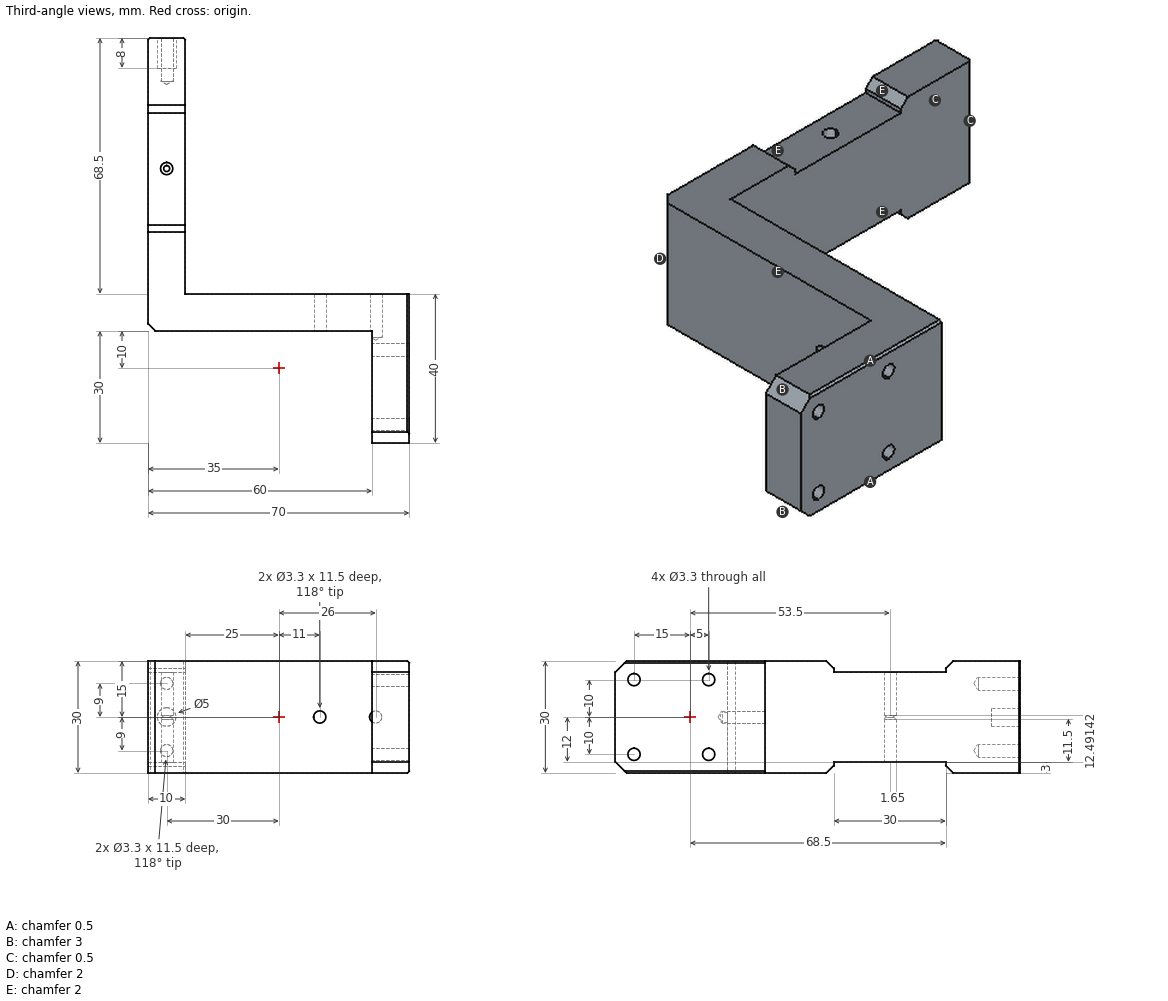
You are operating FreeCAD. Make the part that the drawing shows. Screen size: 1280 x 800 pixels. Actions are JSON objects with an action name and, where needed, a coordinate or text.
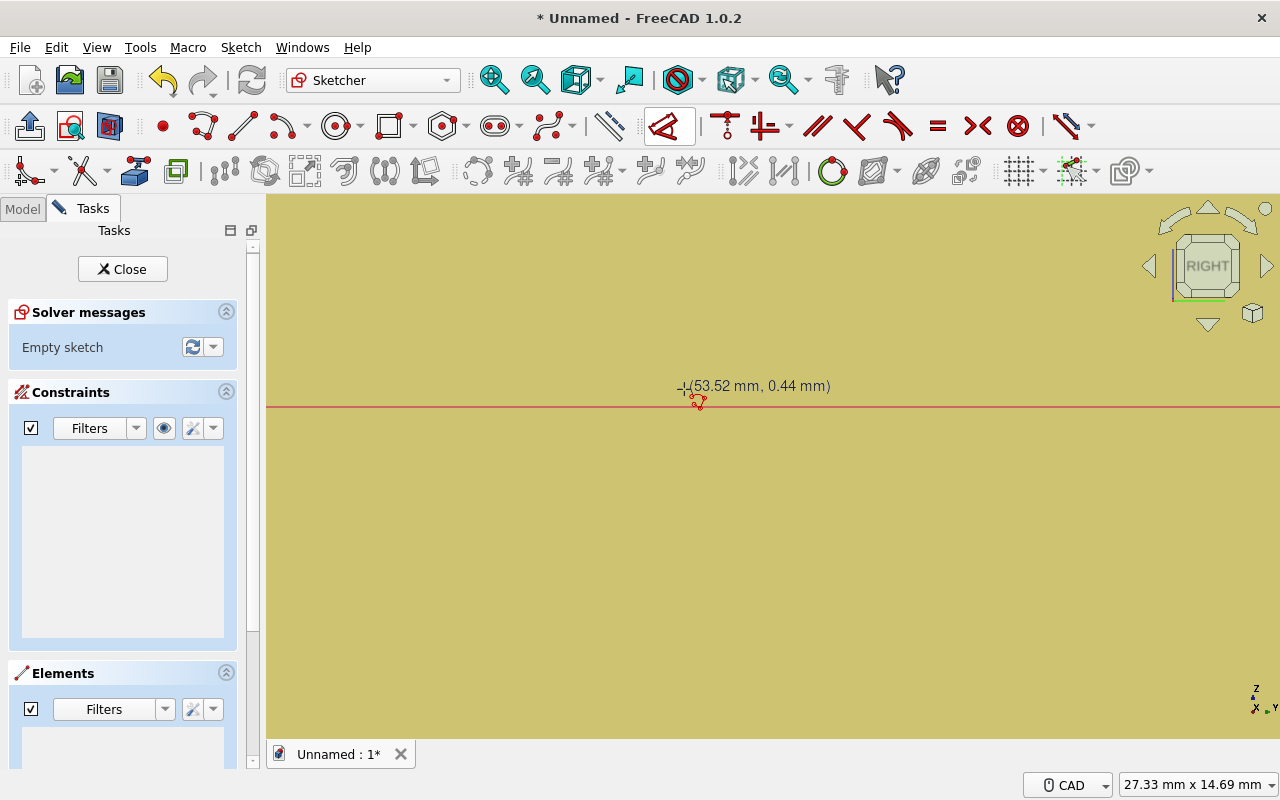
{"action": "scroll", "coordinate": [692, 392], "scroll_direction": "down", "scroll_amount": 3}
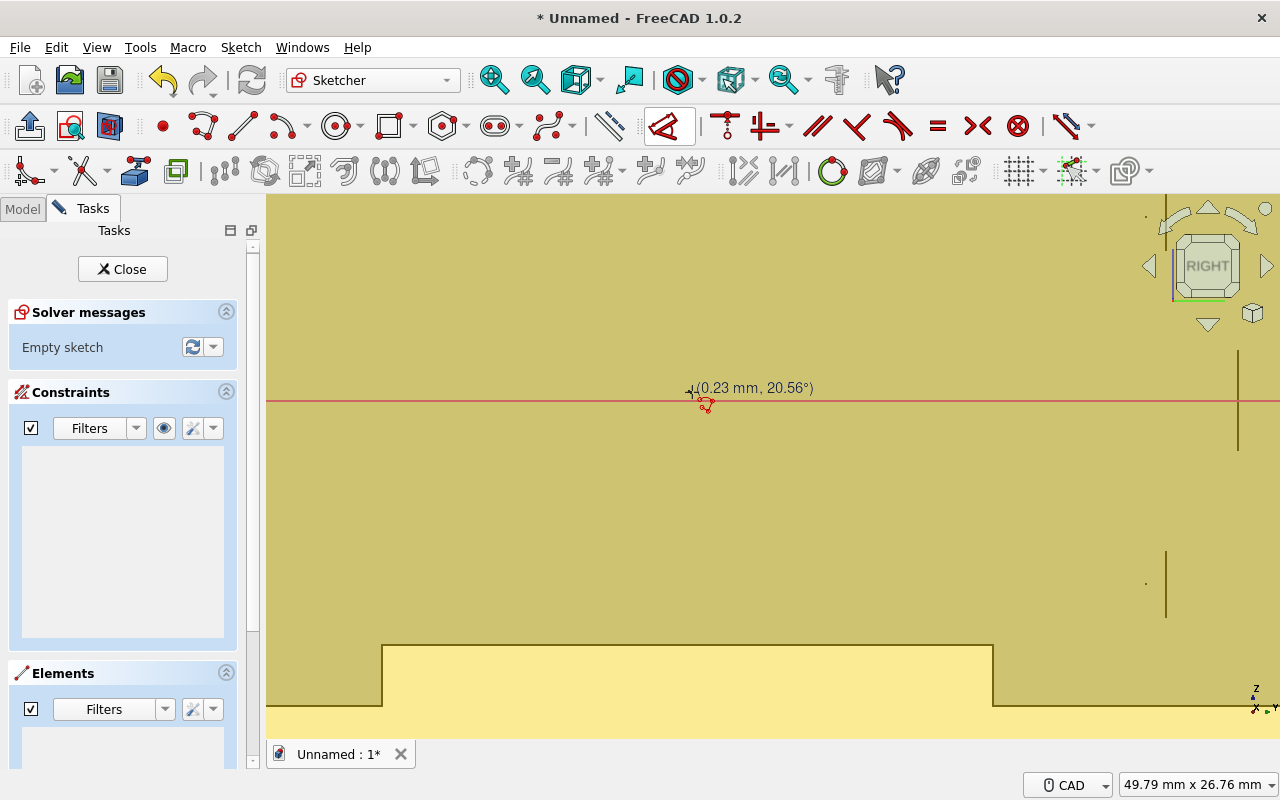
{"action": "left_click", "coordinate": [688, 645]}
{"action": "left_click", "coordinate": [721, 645]}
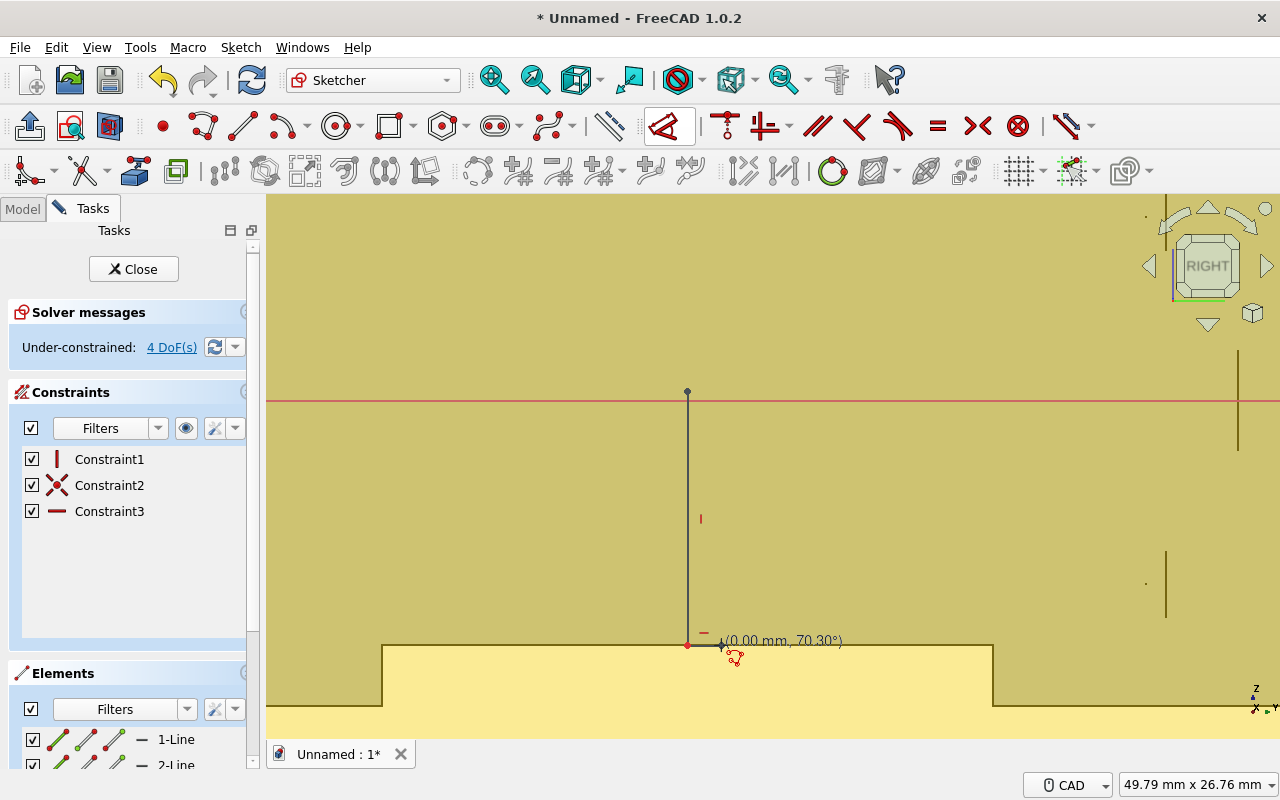
{"action": "scroll", "coordinate": [721, 411], "scroll_direction": "up", "scroll_amount": 3}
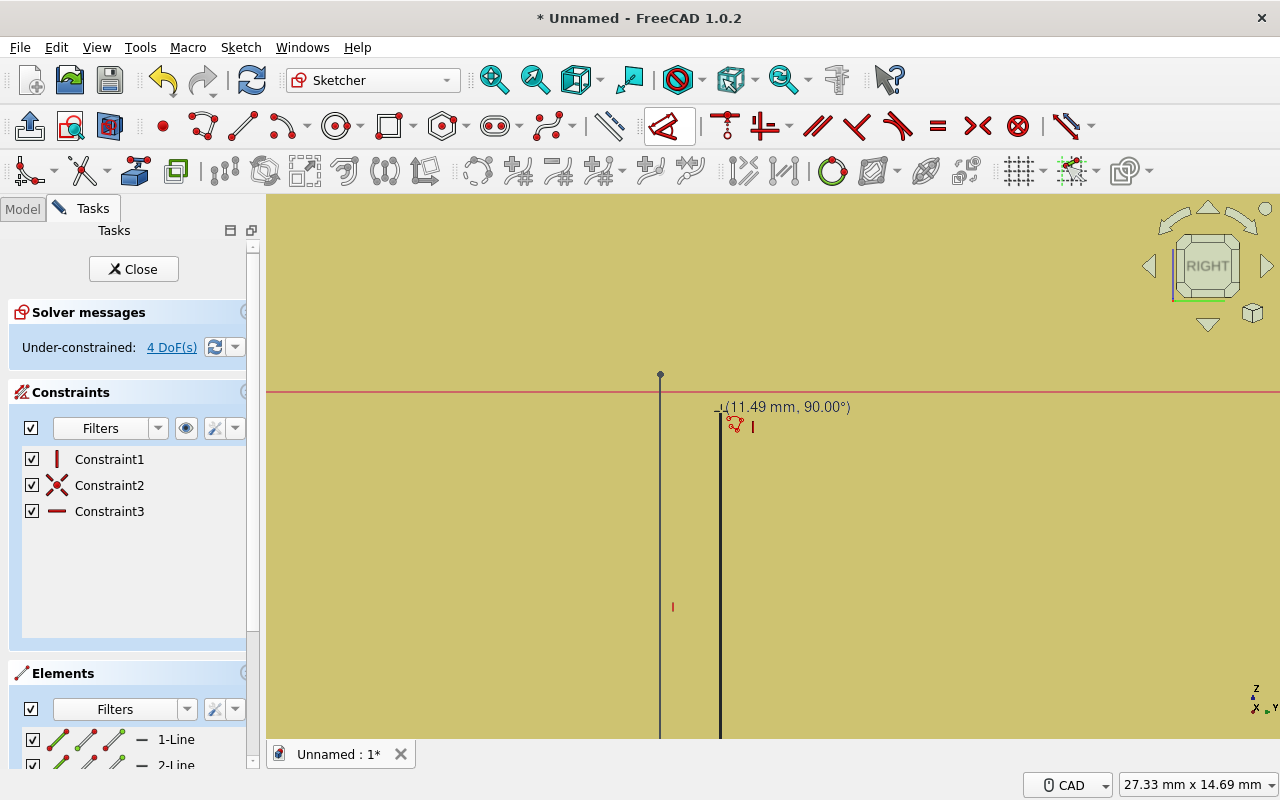
{"action": "left_click", "coordinate": [721, 410]}
{"action": "left_click", "coordinate": [660, 374]}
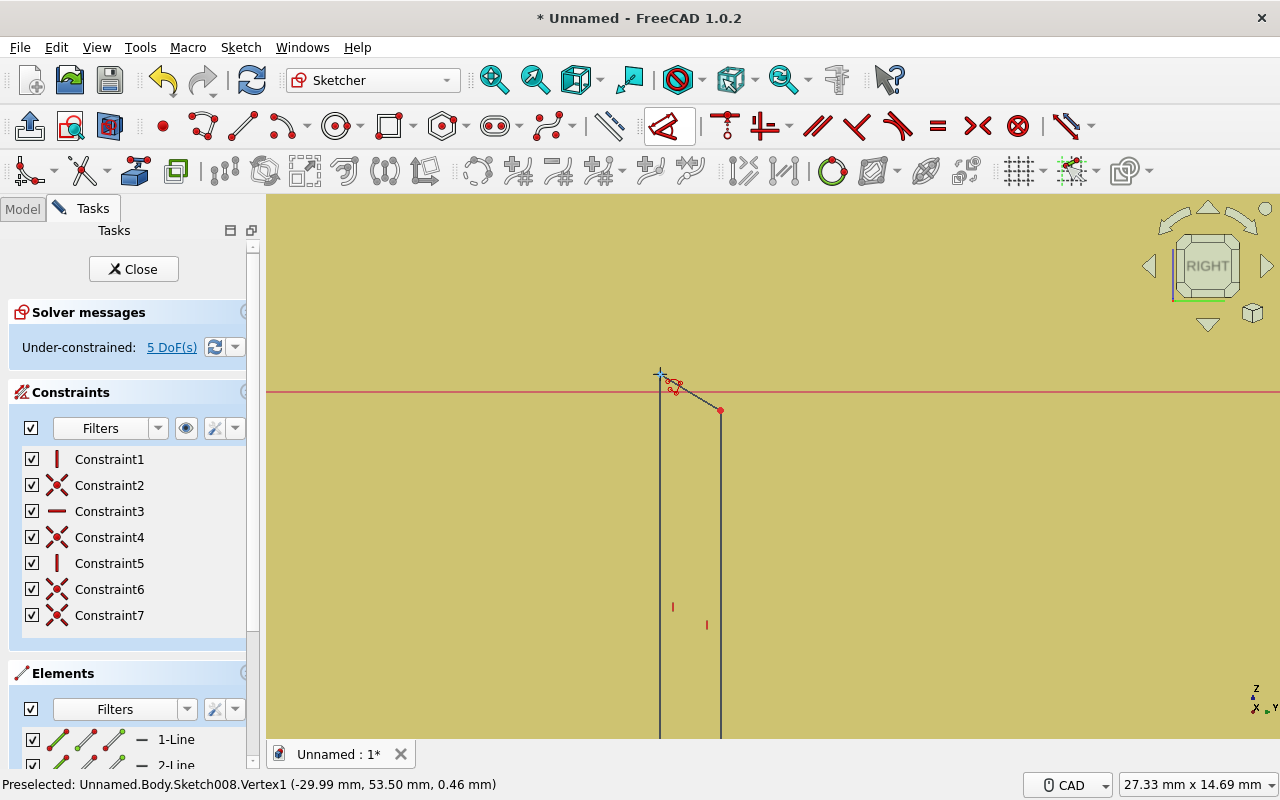
{"action": "left_click", "coordinate": [244, 126]}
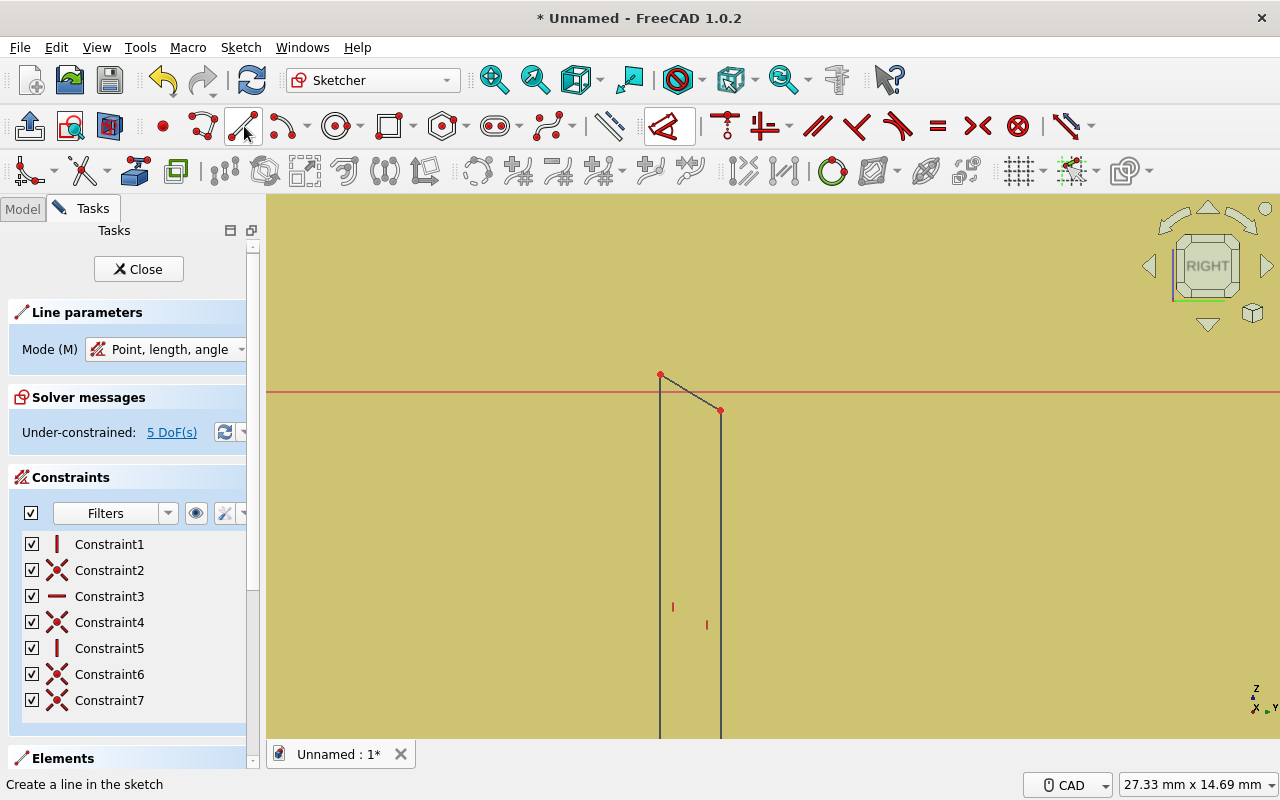
{"action": "left_click", "coordinate": [660, 327]}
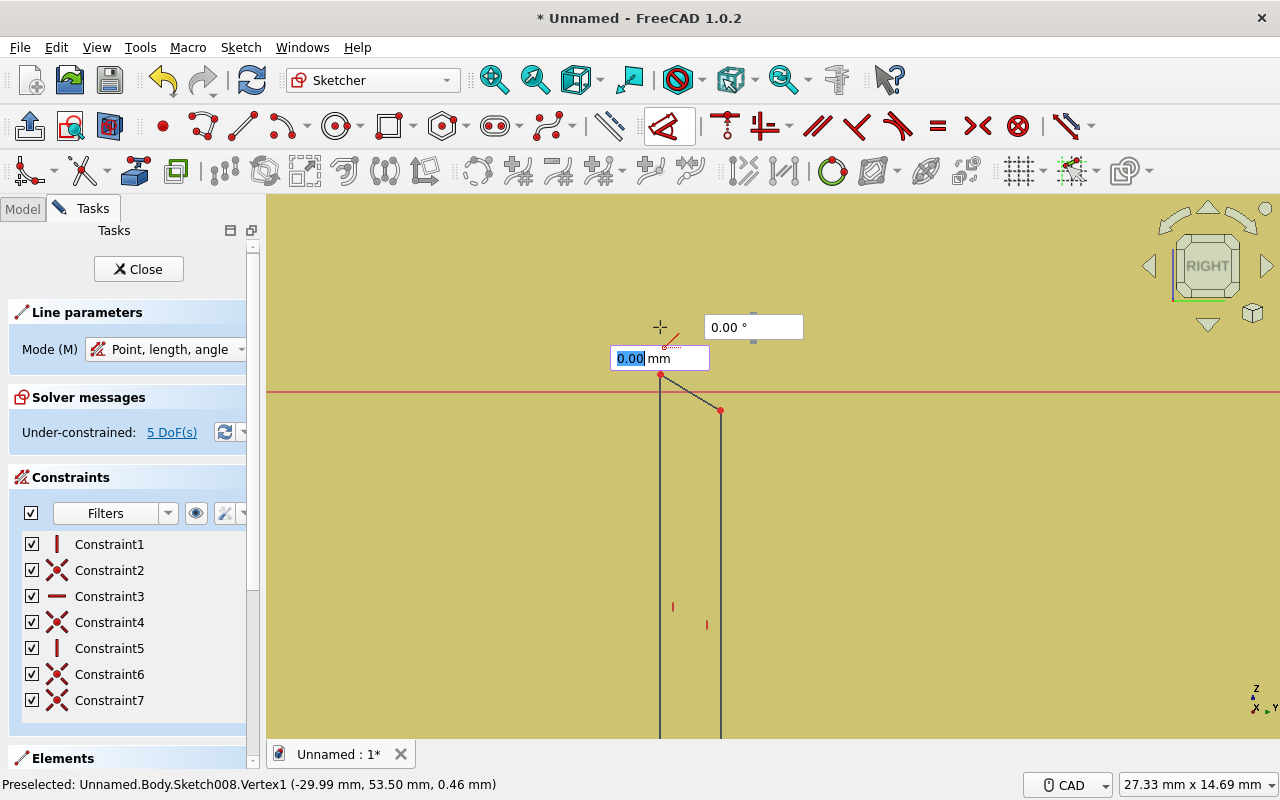
{"action": "scroll", "coordinate": [721, 411], "scroll_direction": "down", "scroll_amount": 3}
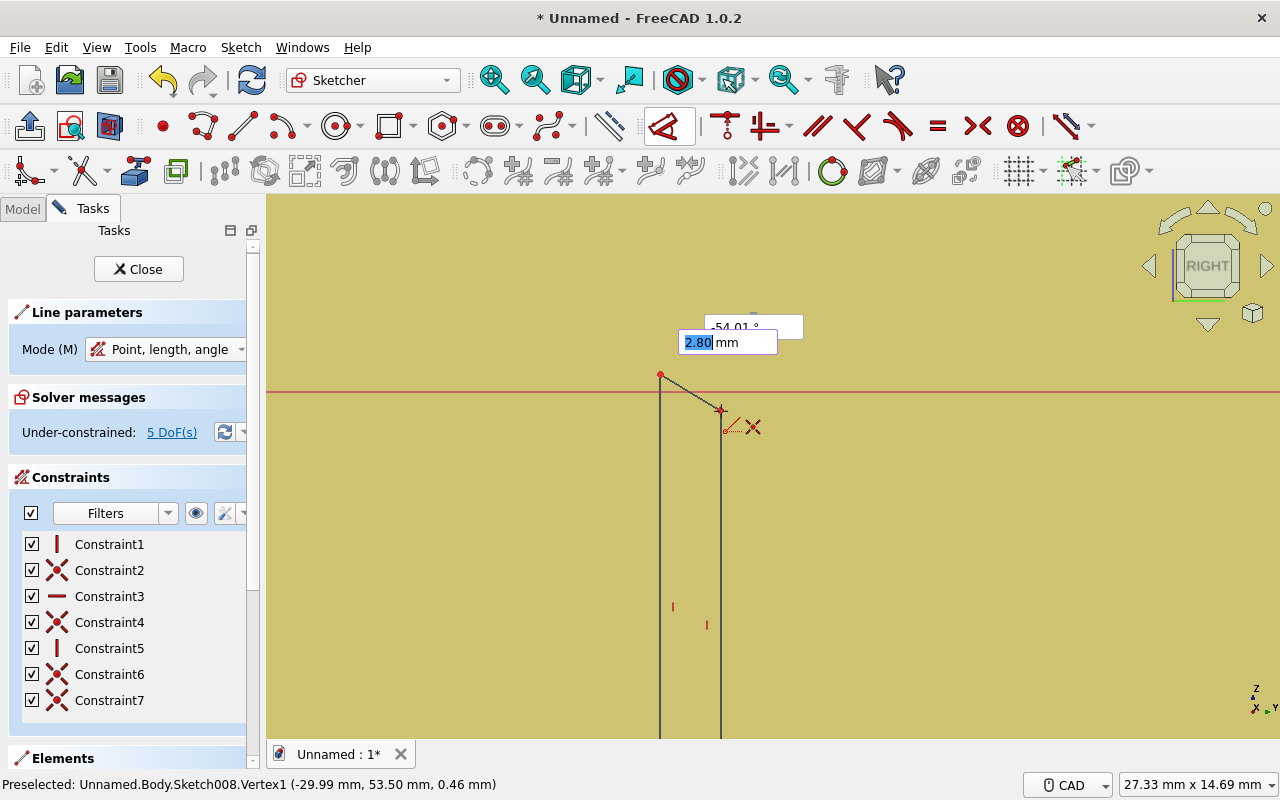
{"action": "left_click", "coordinate": [688, 289]}
{"action": "key", "text": "Escape"}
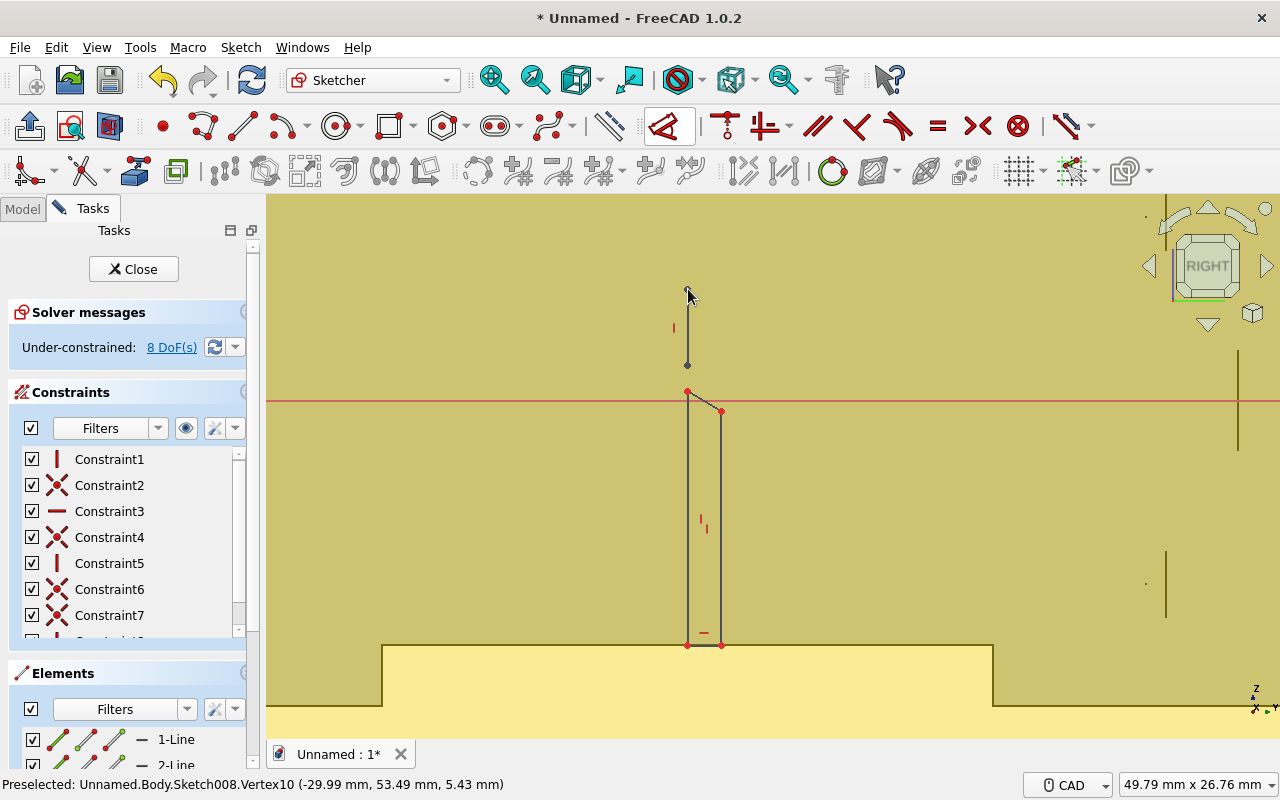
{"action": "left_click", "coordinate": [688, 343]}